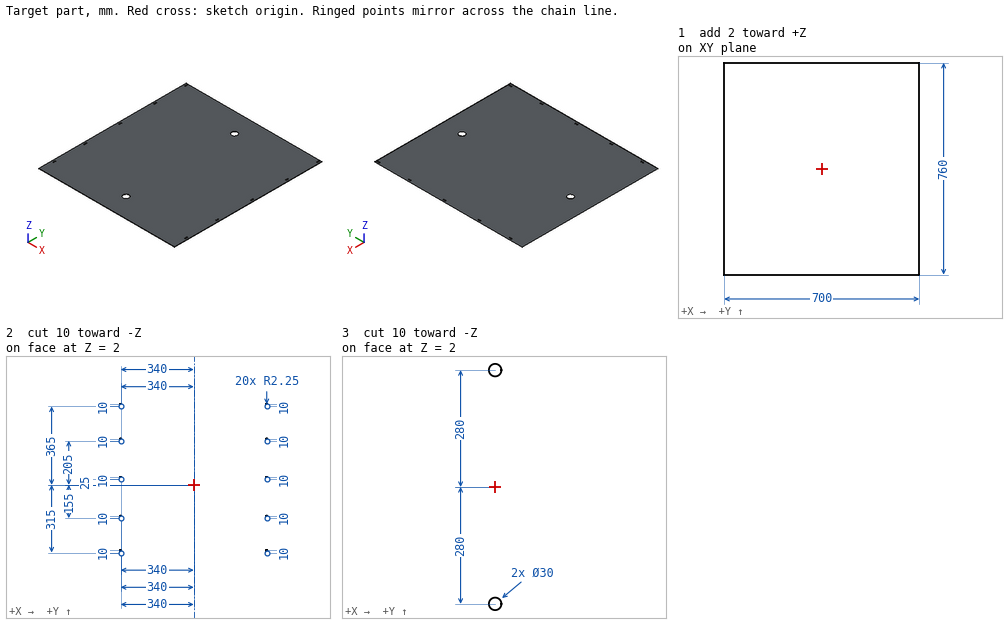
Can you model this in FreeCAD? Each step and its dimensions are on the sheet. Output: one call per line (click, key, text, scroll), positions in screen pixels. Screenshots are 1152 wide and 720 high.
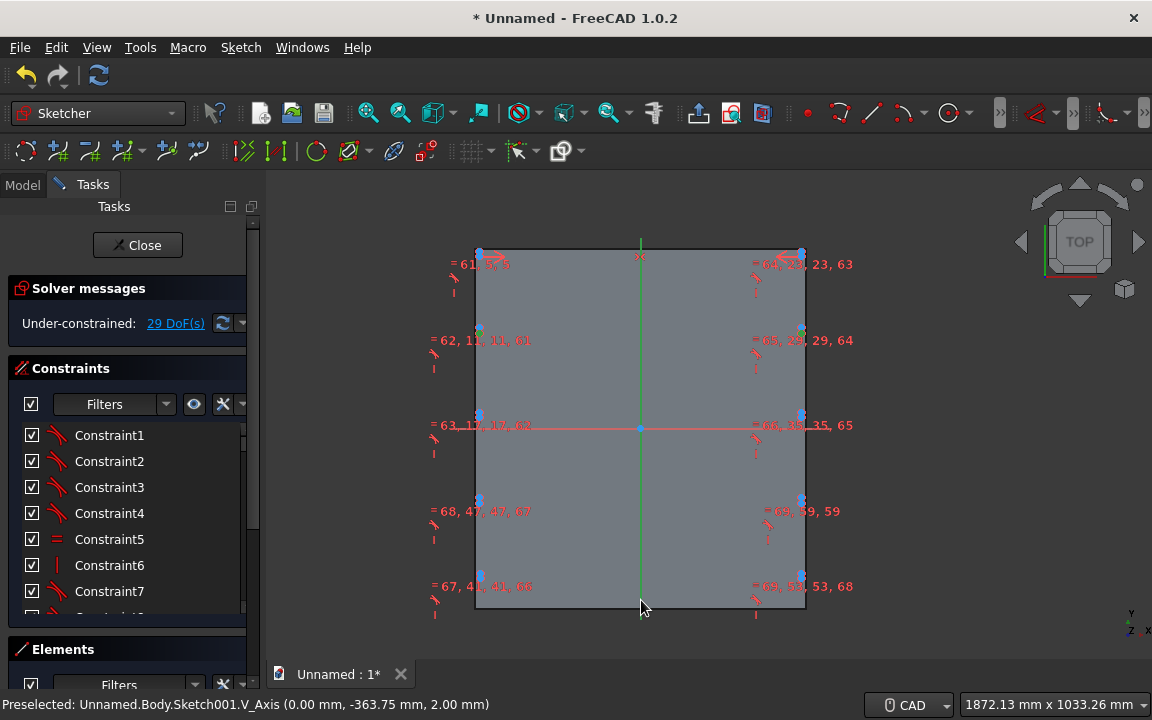
key(s)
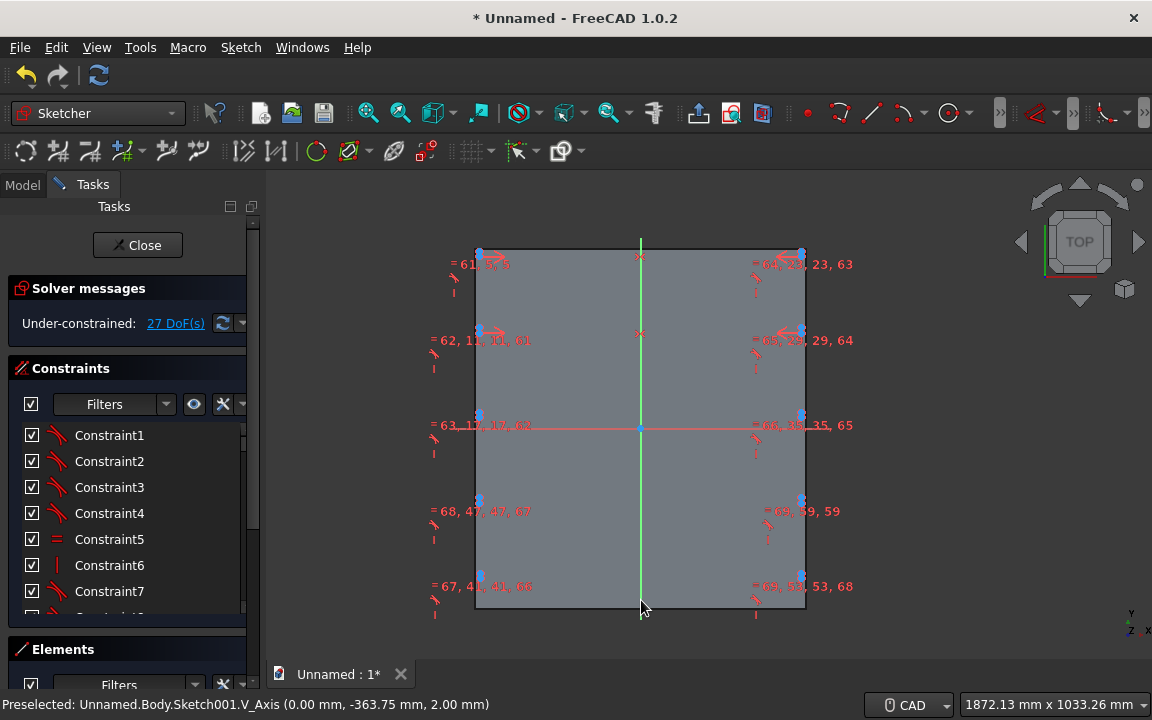
scroll(480, 418, up, 13)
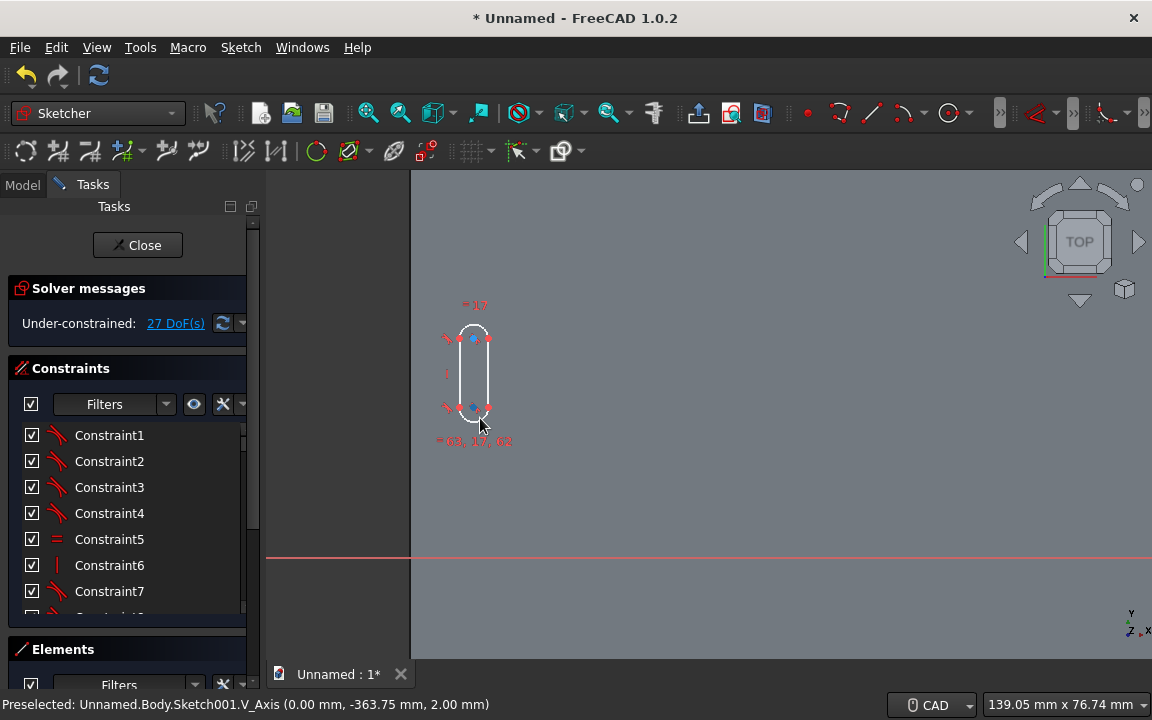
click(474, 408)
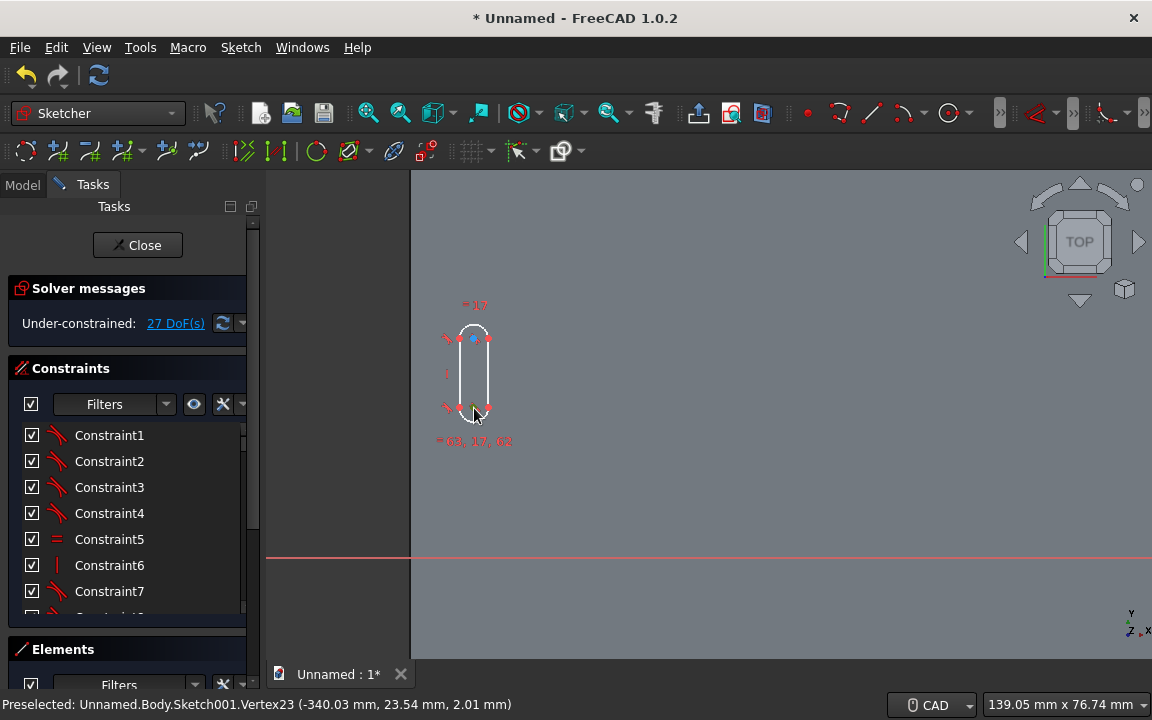
scroll(480, 418, down, 13)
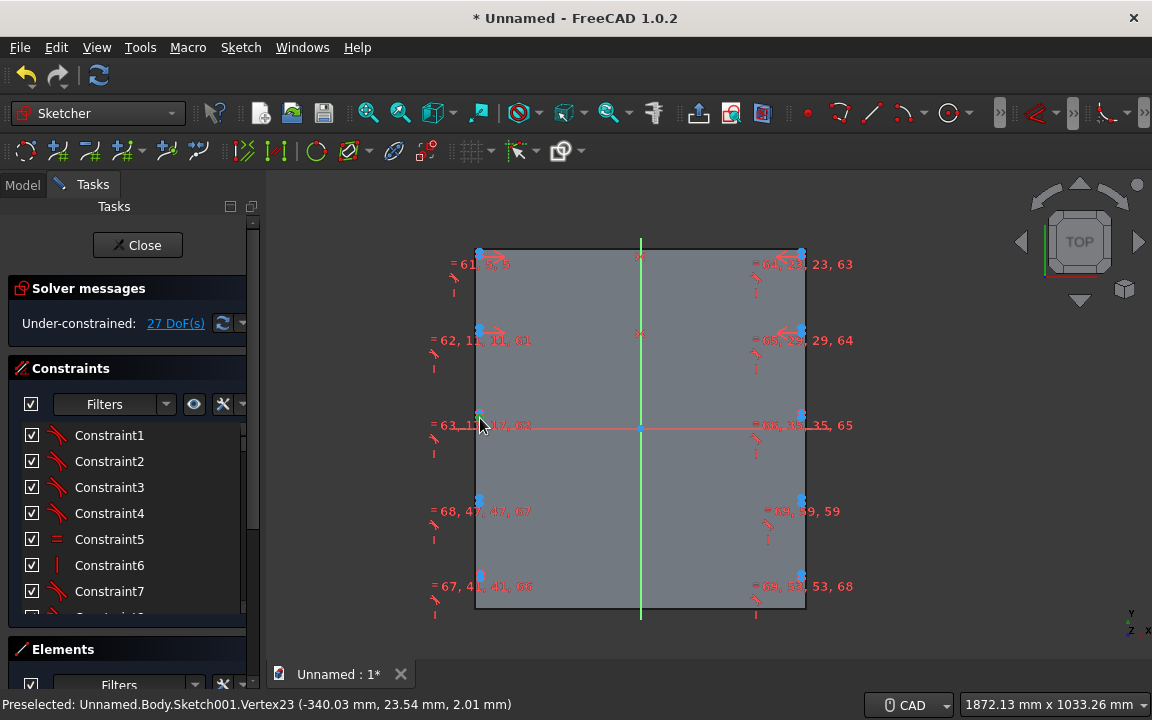
scroll(802, 418, up, 13)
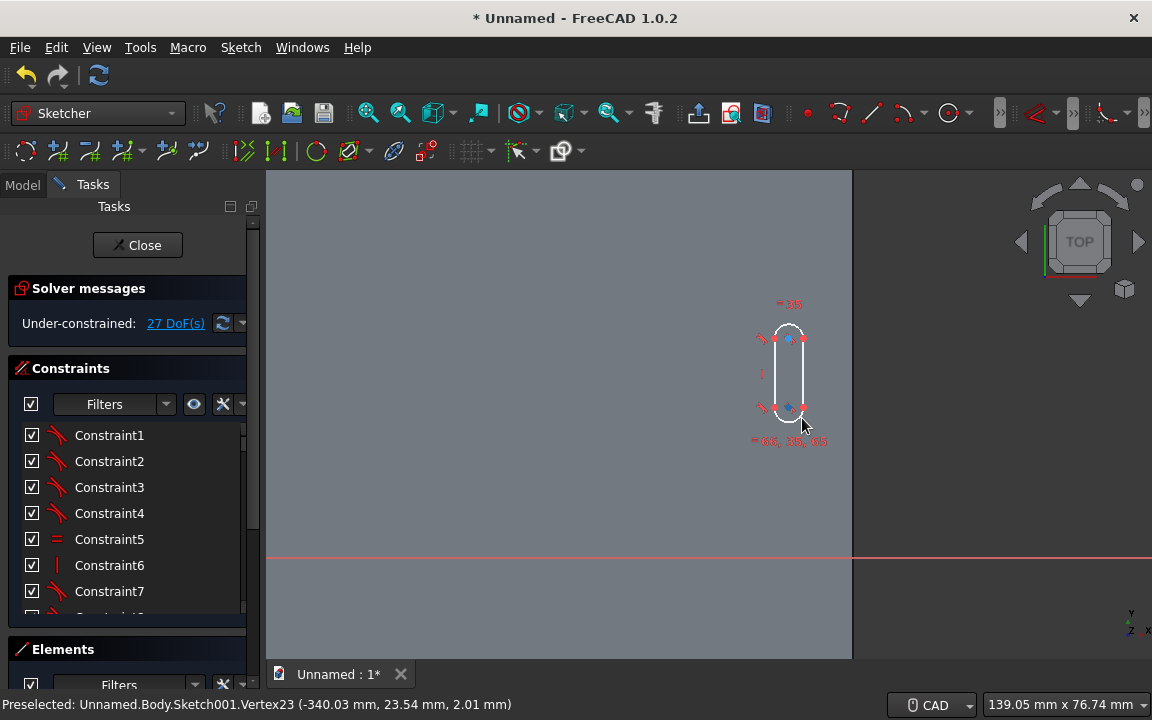
click(789, 408)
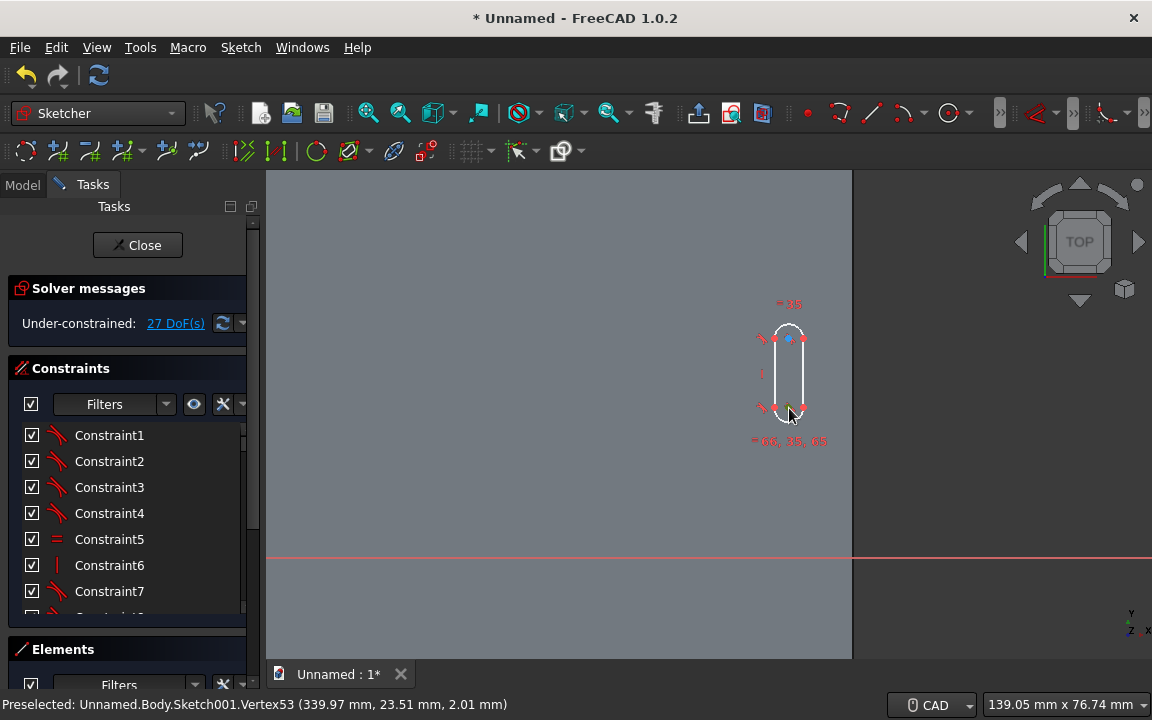
scroll(802, 418, down, 13)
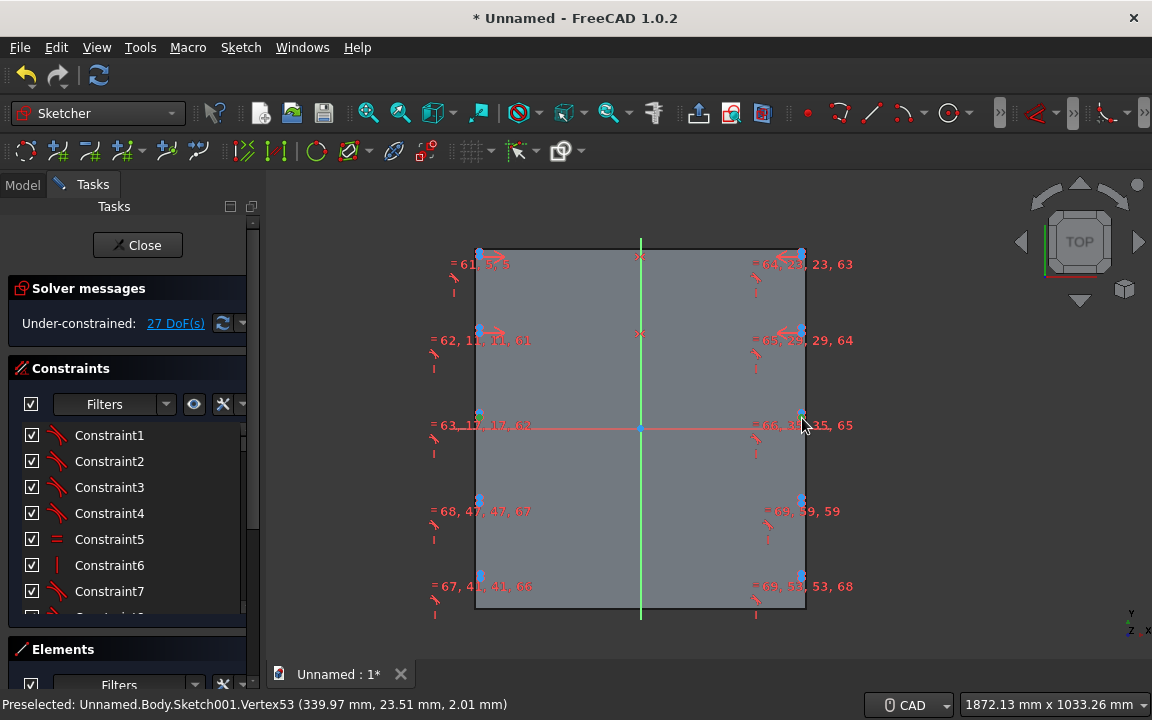
click(641, 600)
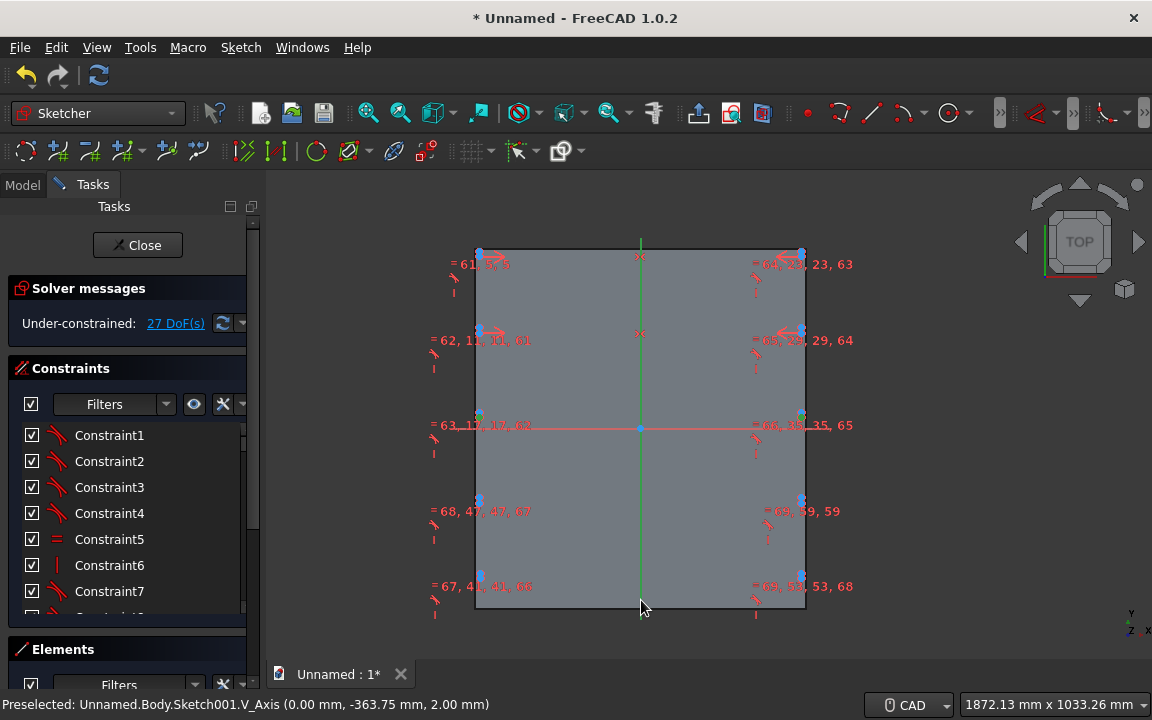
key(s)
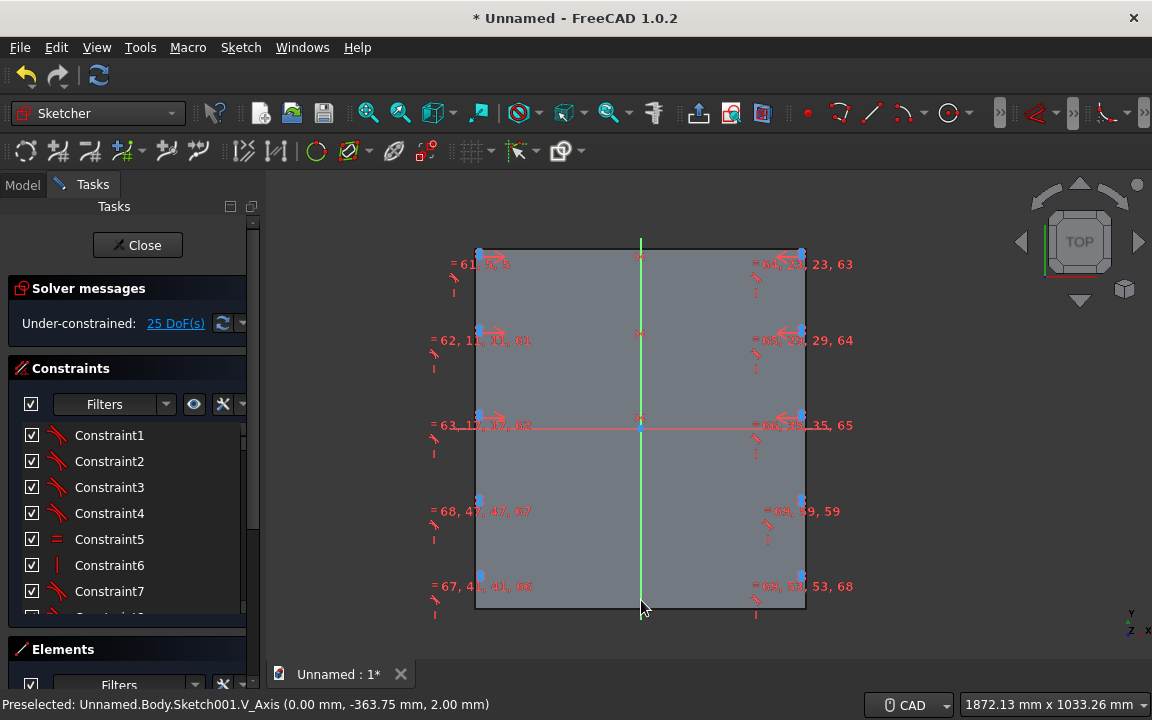
scroll(480, 579, up, 13)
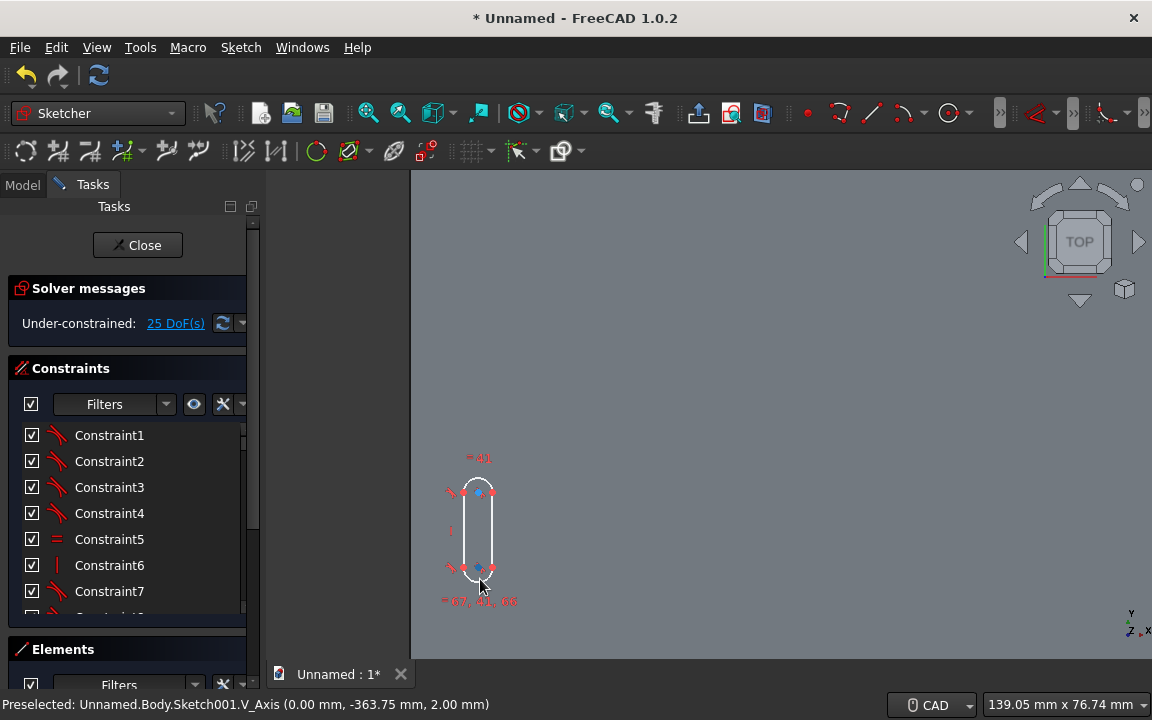
click(478, 568)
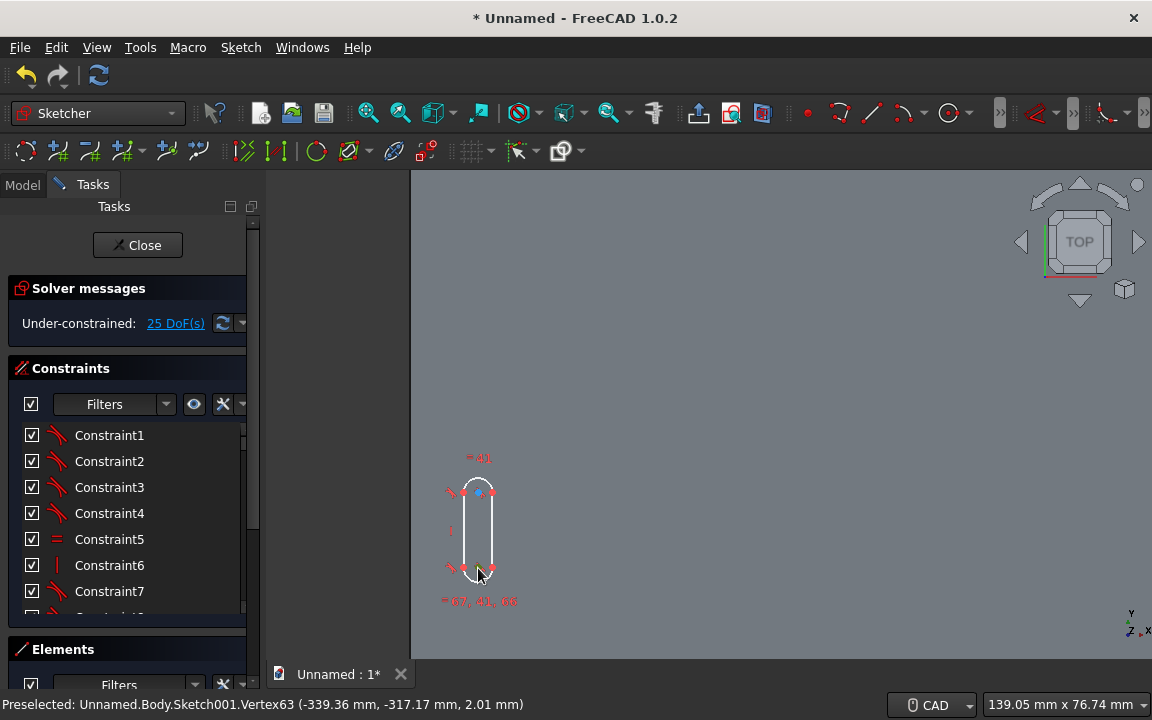
scroll(480, 580, down, 13)